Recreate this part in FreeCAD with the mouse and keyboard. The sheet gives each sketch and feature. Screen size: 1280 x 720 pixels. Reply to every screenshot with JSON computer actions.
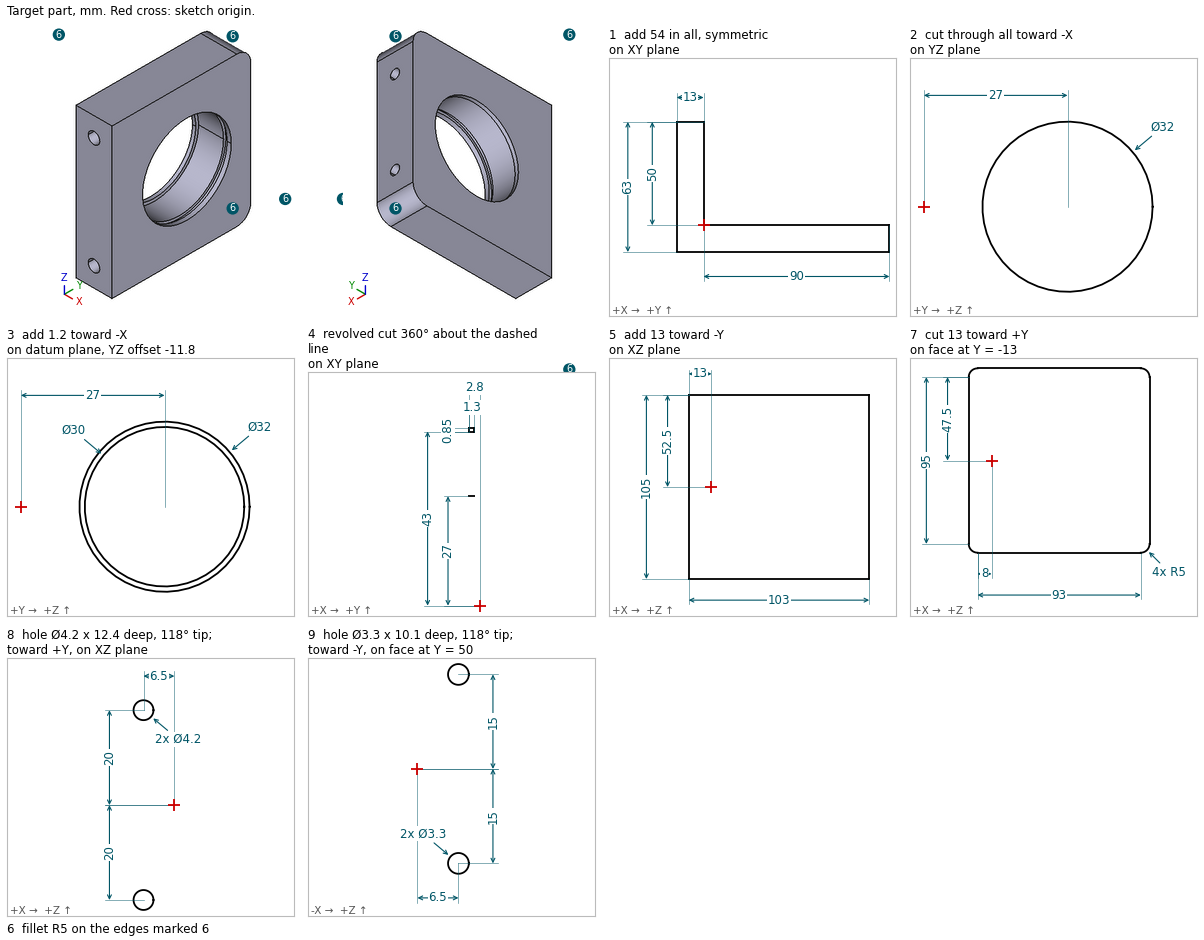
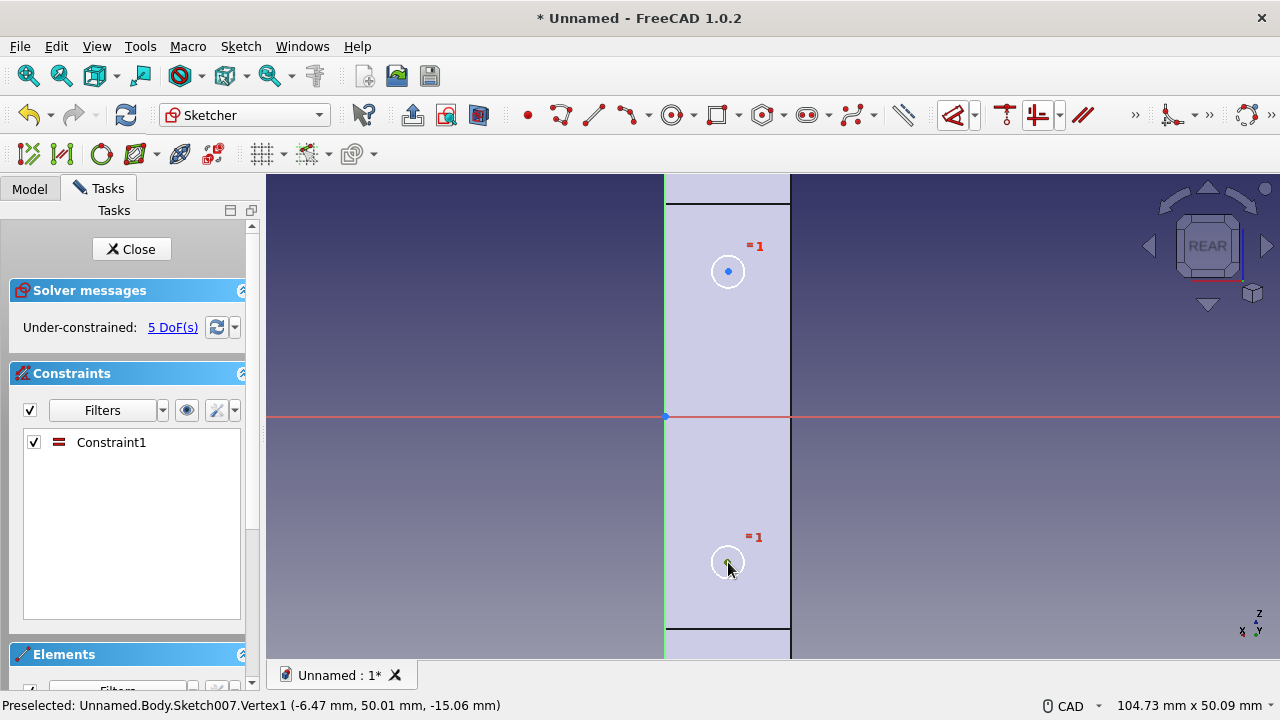
{"action": "left_click", "coordinate": [728, 272]}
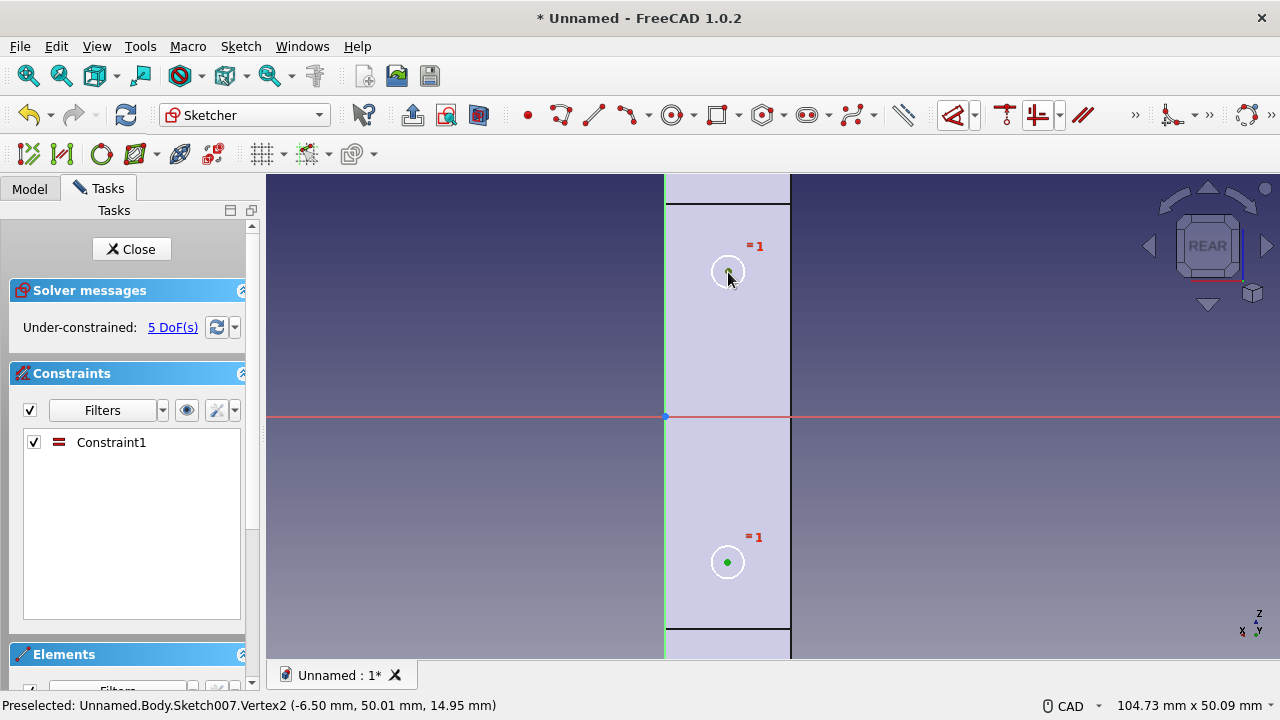
{"action": "left_click", "coordinate": [1060, 116]}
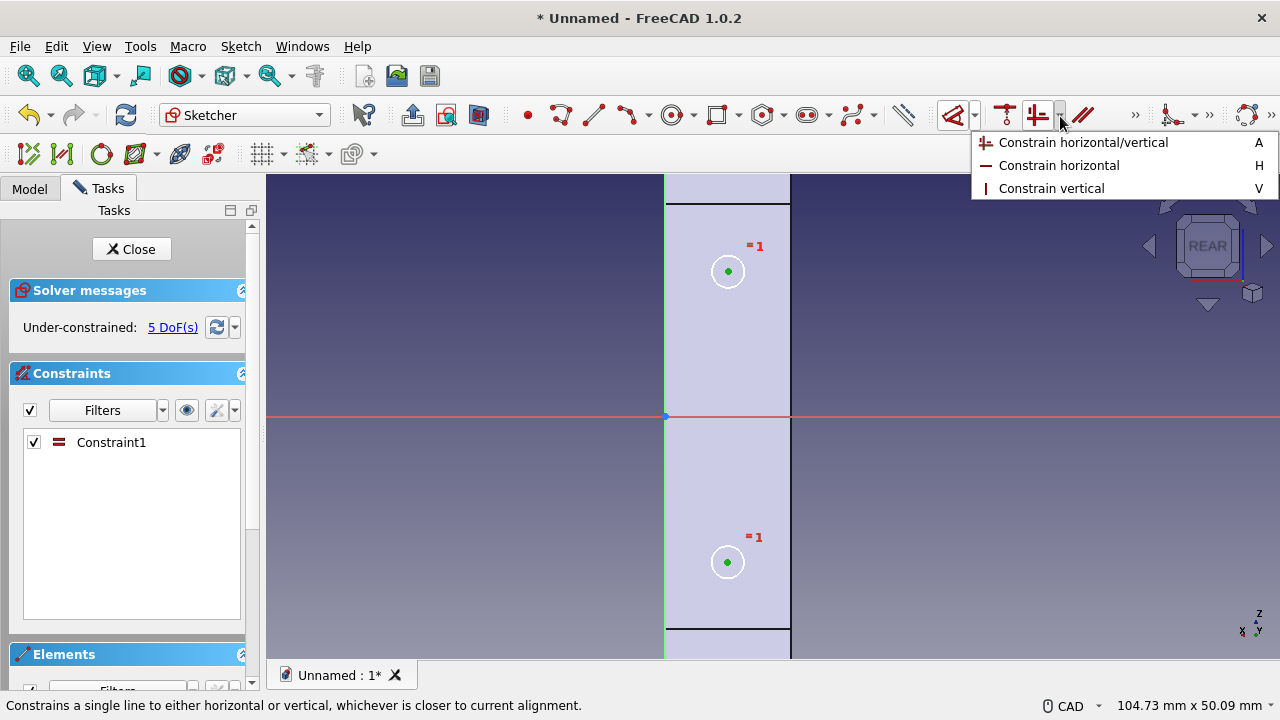
{"action": "left_click", "coordinate": [1125, 188]}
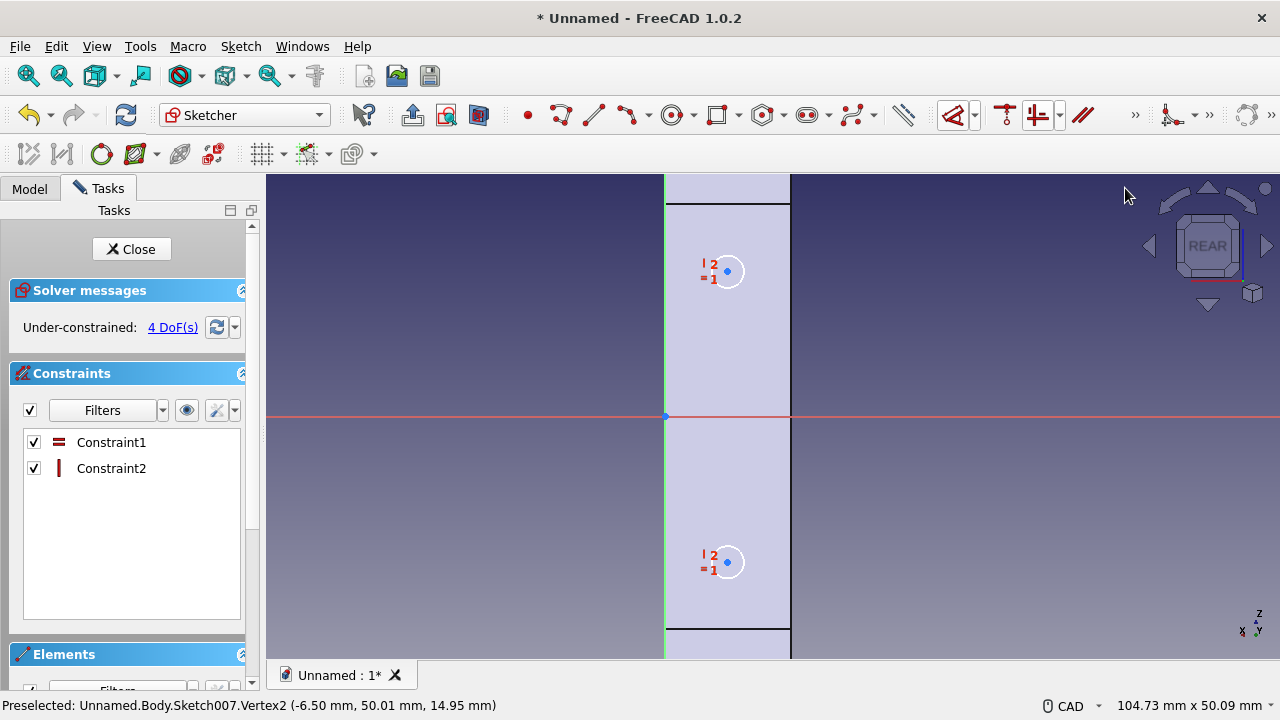
{"action": "scroll", "coordinate": [739, 551], "scroll_direction": "up", "scroll_amount": 2}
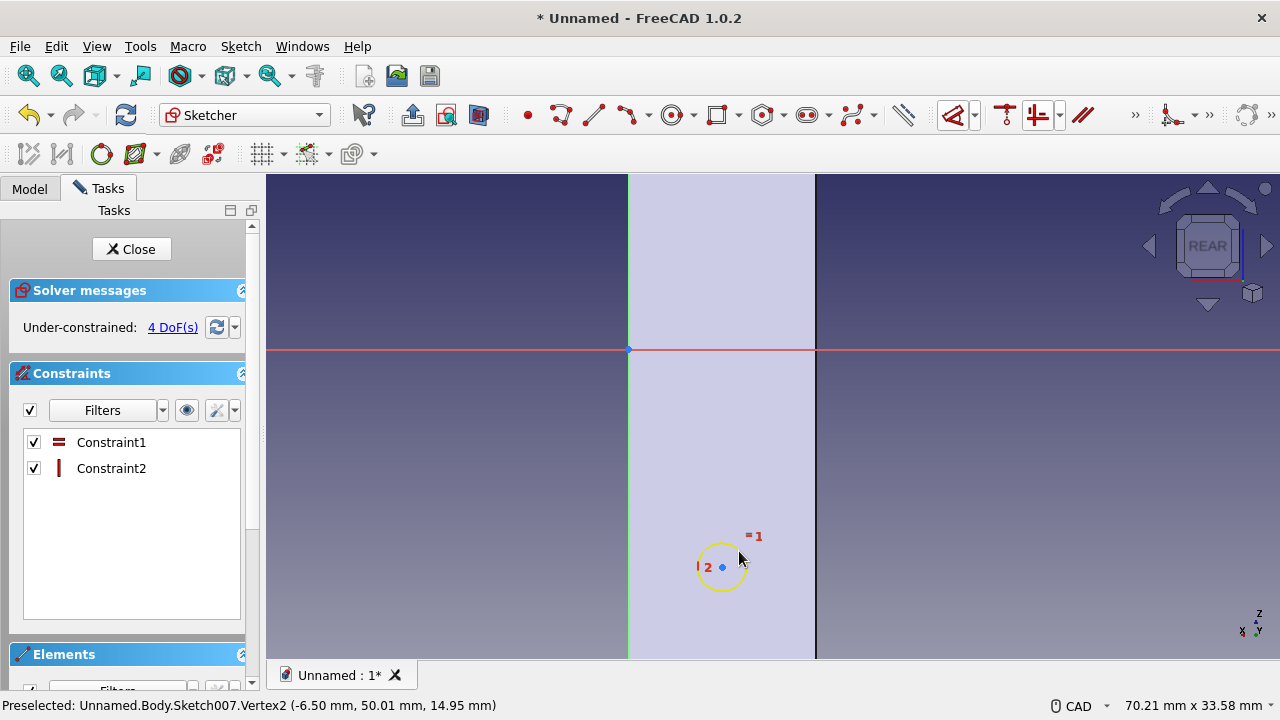
{"action": "left_click", "coordinate": [739, 550]}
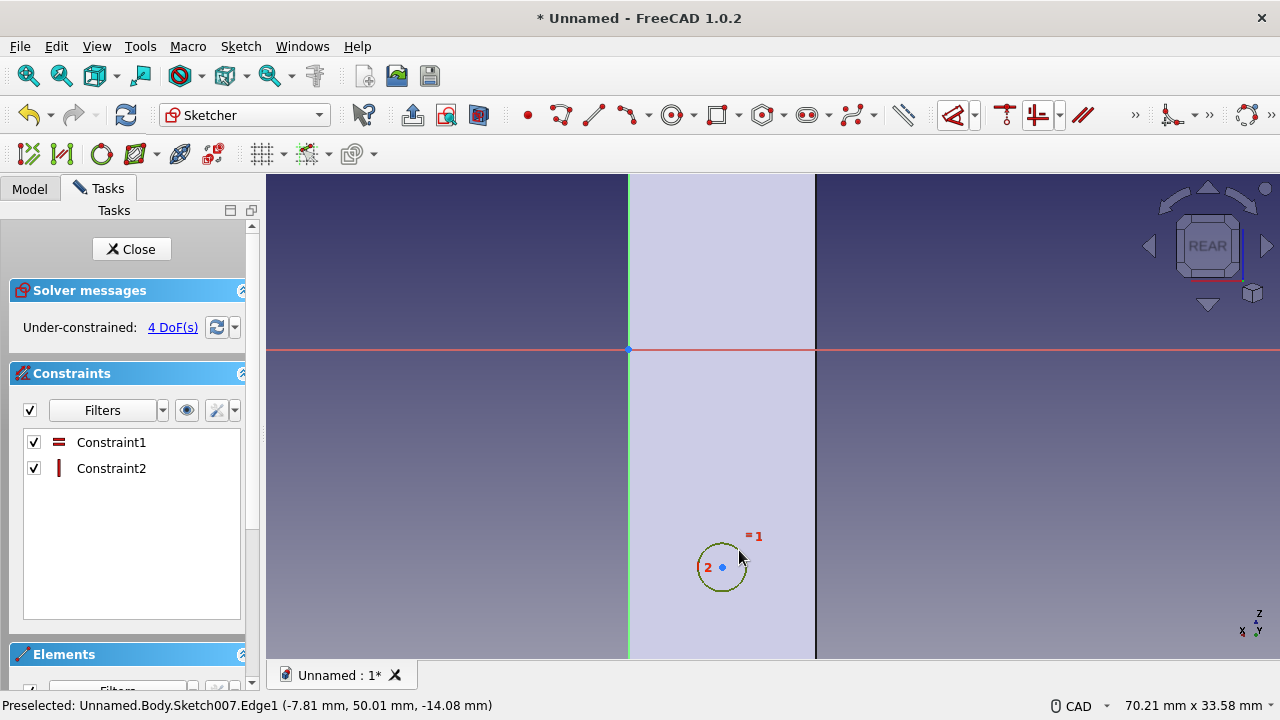
{"action": "left_click", "coordinate": [974, 116]}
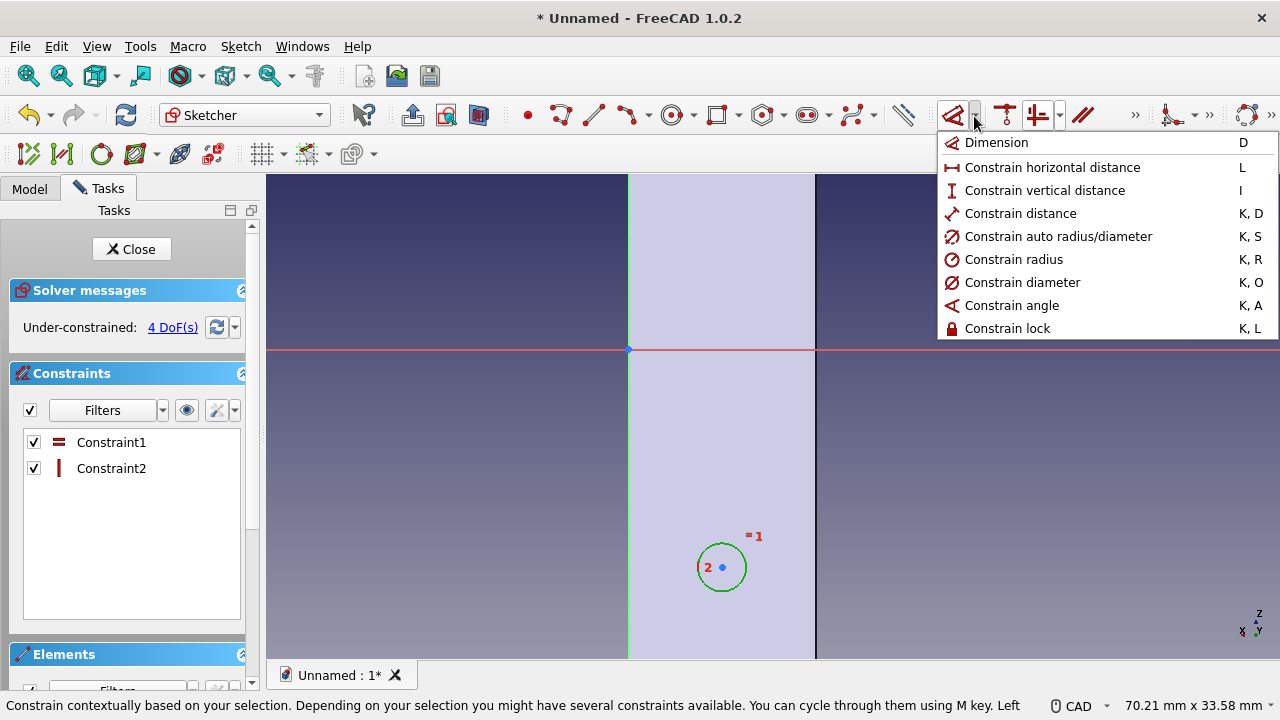
{"action": "left_click", "coordinate": [1108, 282]}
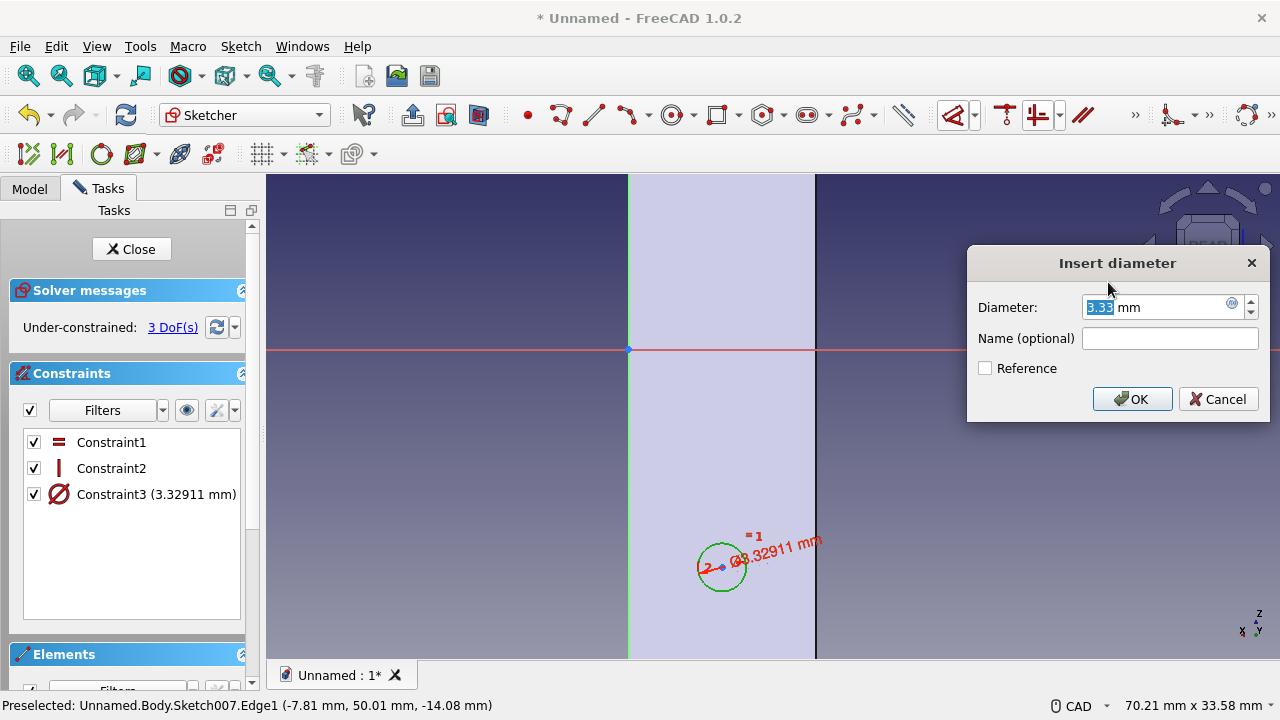
{"action": "type", "text": "3.3"}
{"action": "key", "text": "Return"}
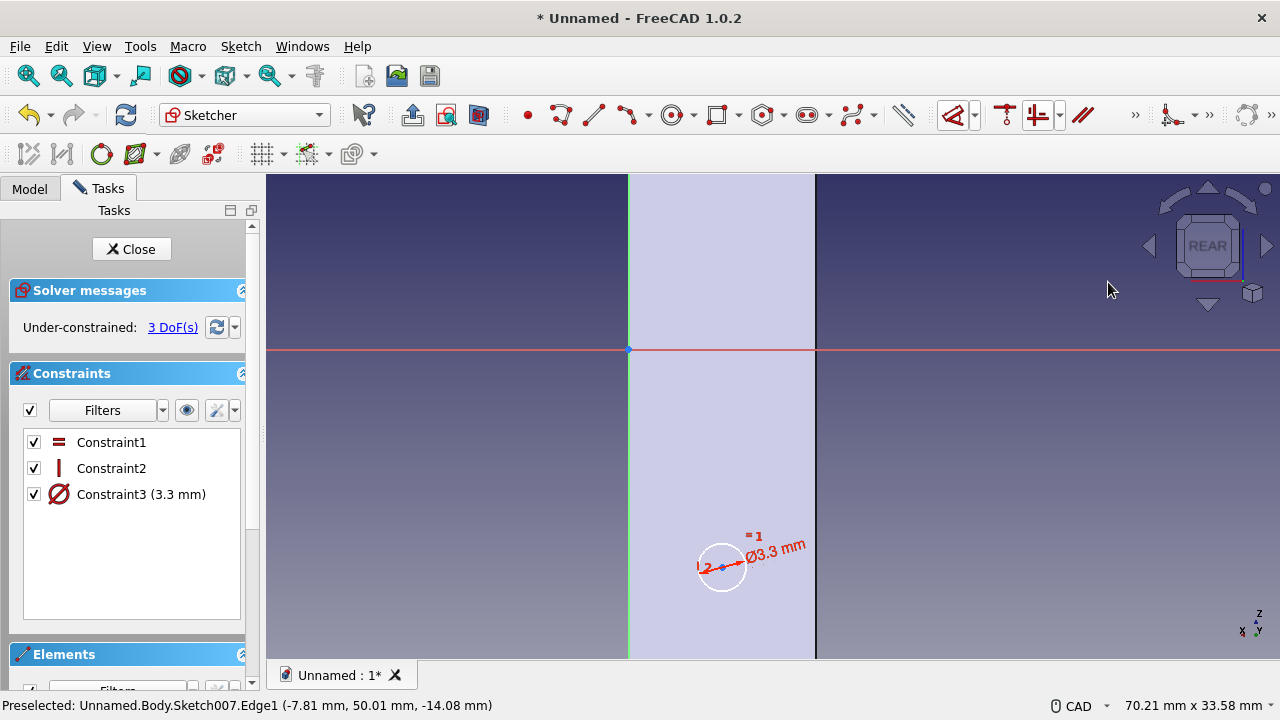
{"action": "left_click", "coordinate": [722, 567]}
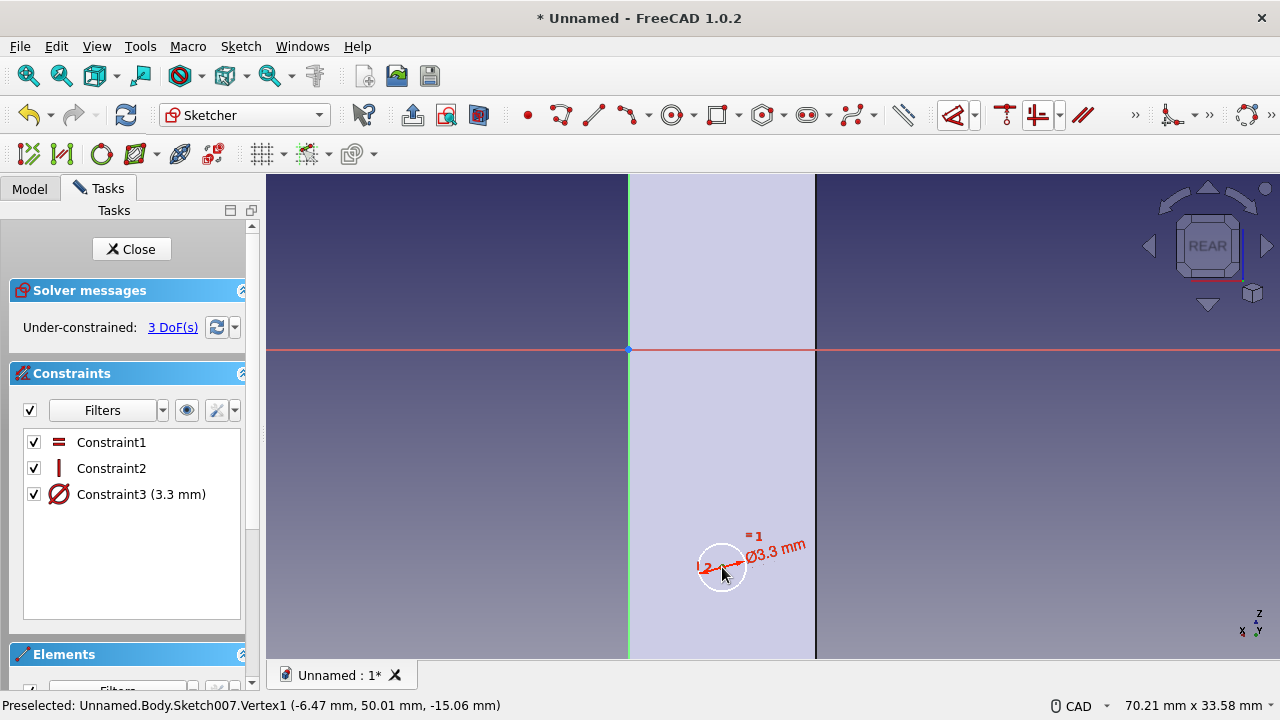
{"action": "left_click", "coordinate": [974, 116]}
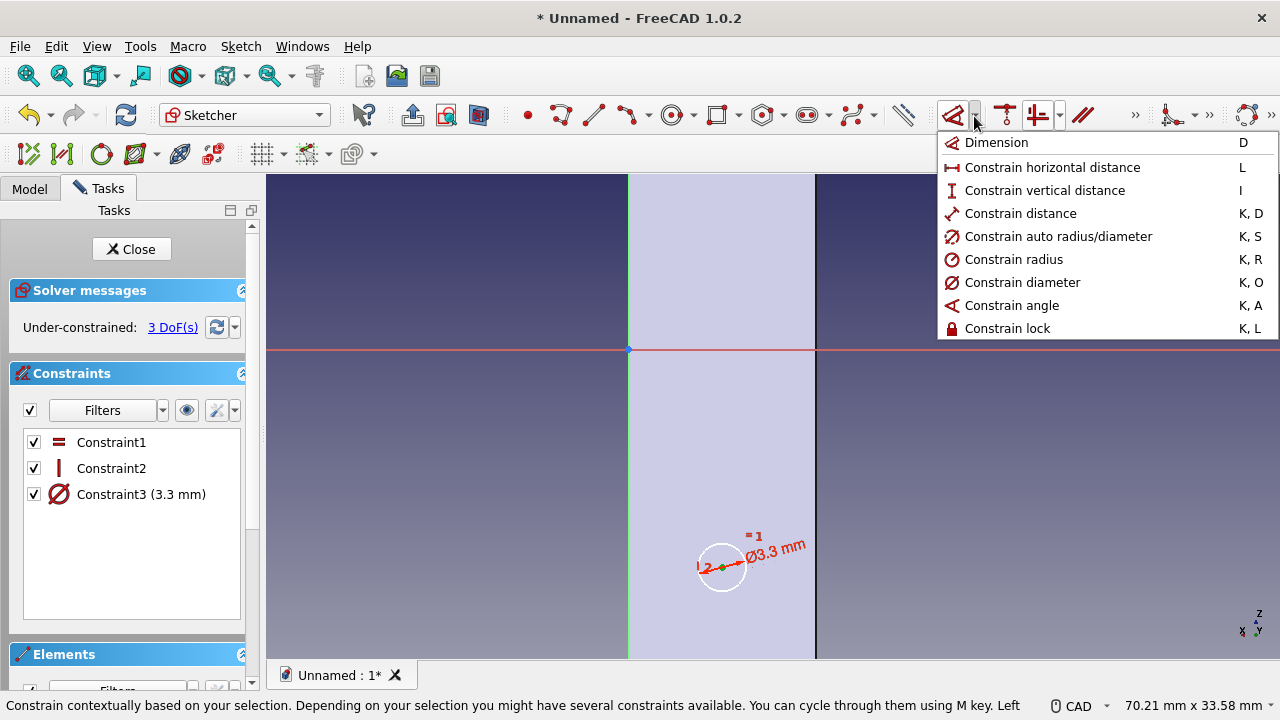
{"action": "left_click", "coordinate": [1108, 190]}